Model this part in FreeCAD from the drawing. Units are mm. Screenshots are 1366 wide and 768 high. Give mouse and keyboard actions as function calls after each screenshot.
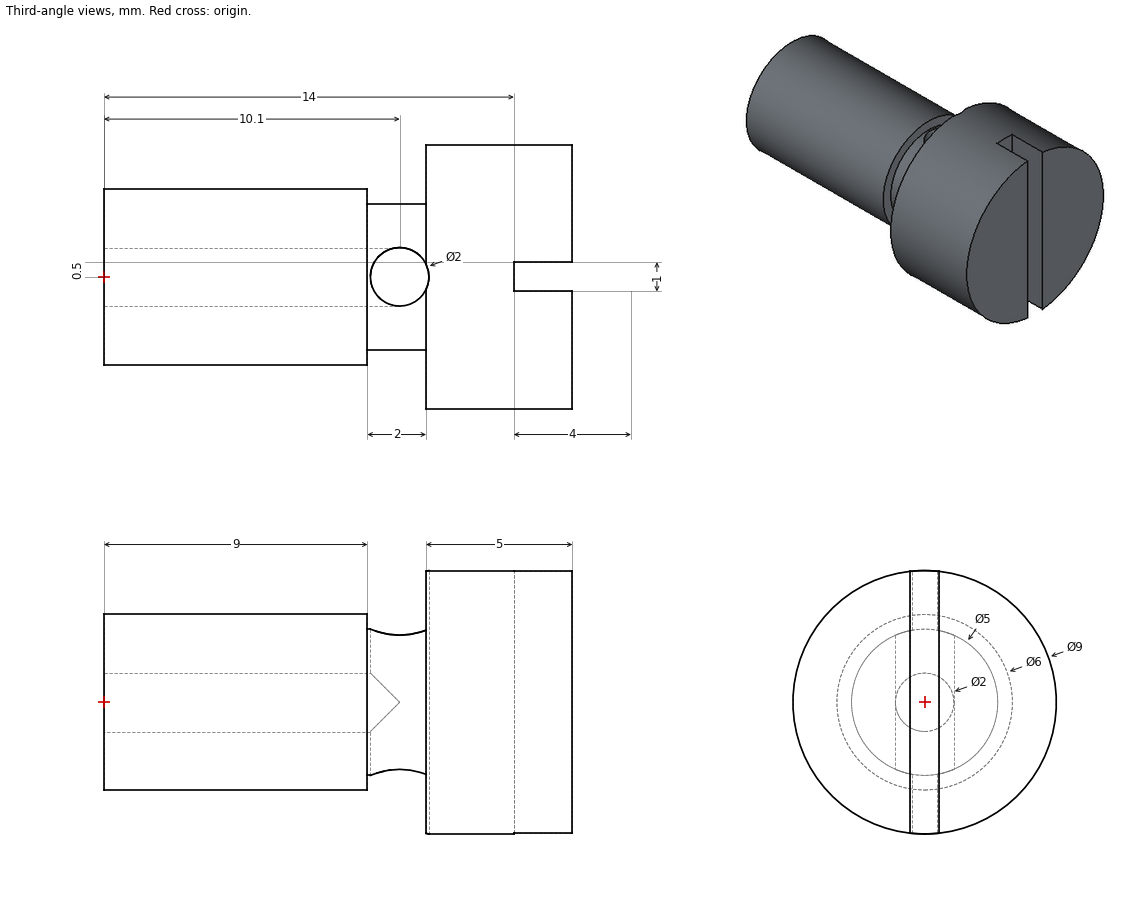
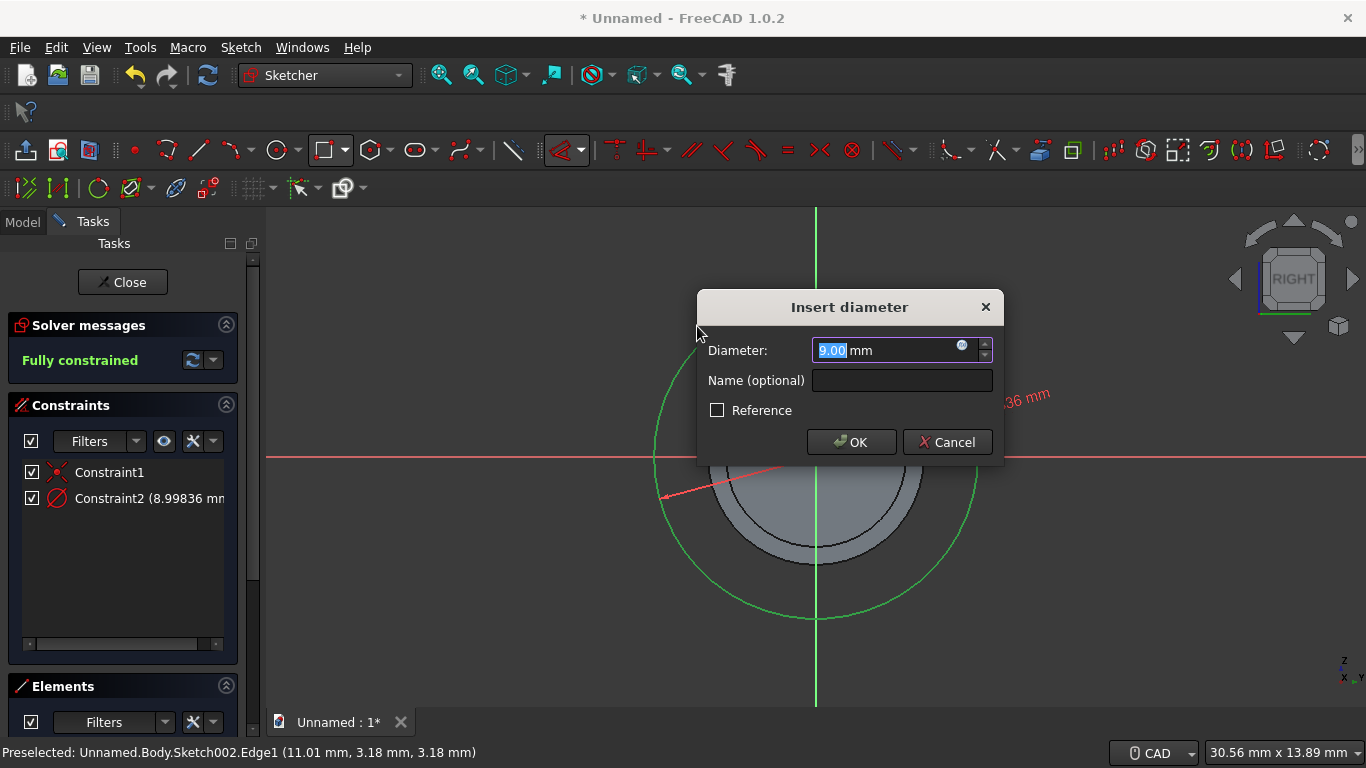
text(9)
key(Return)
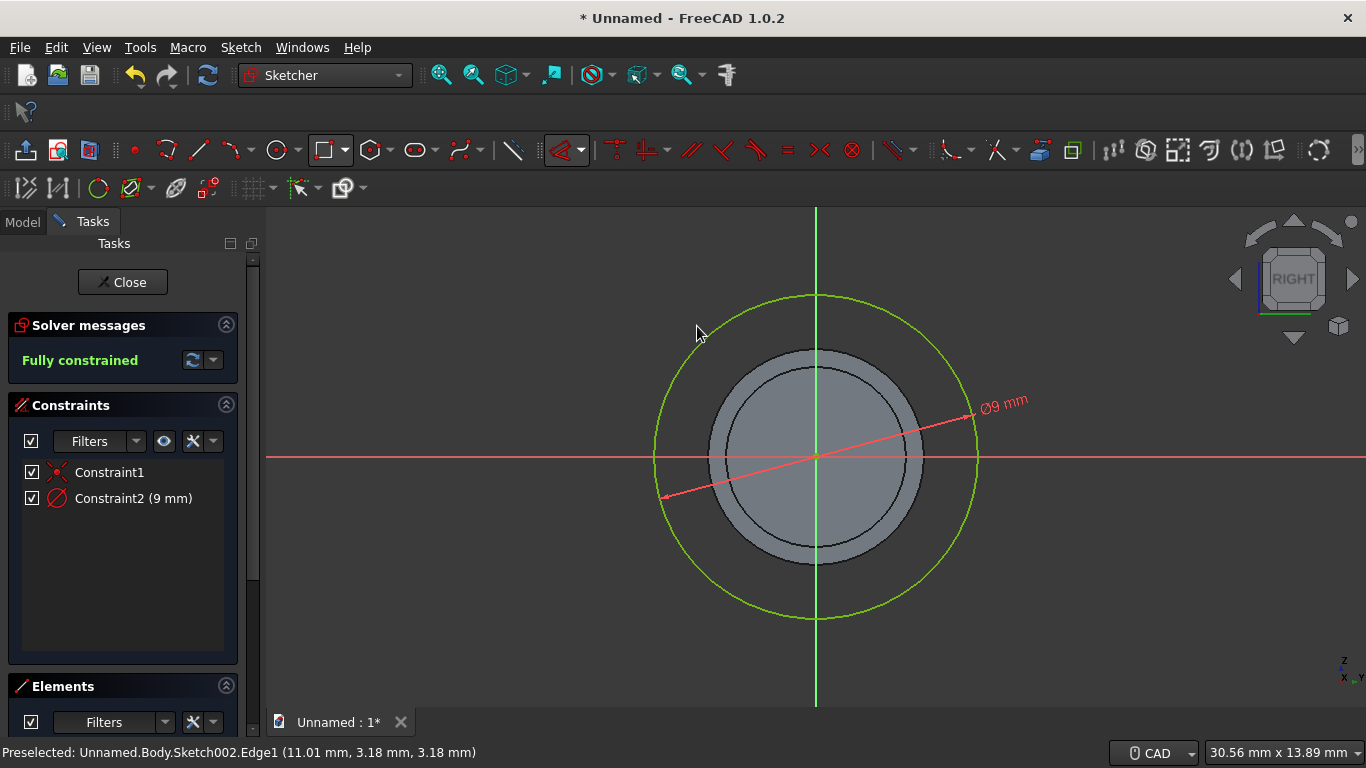
click(123, 282)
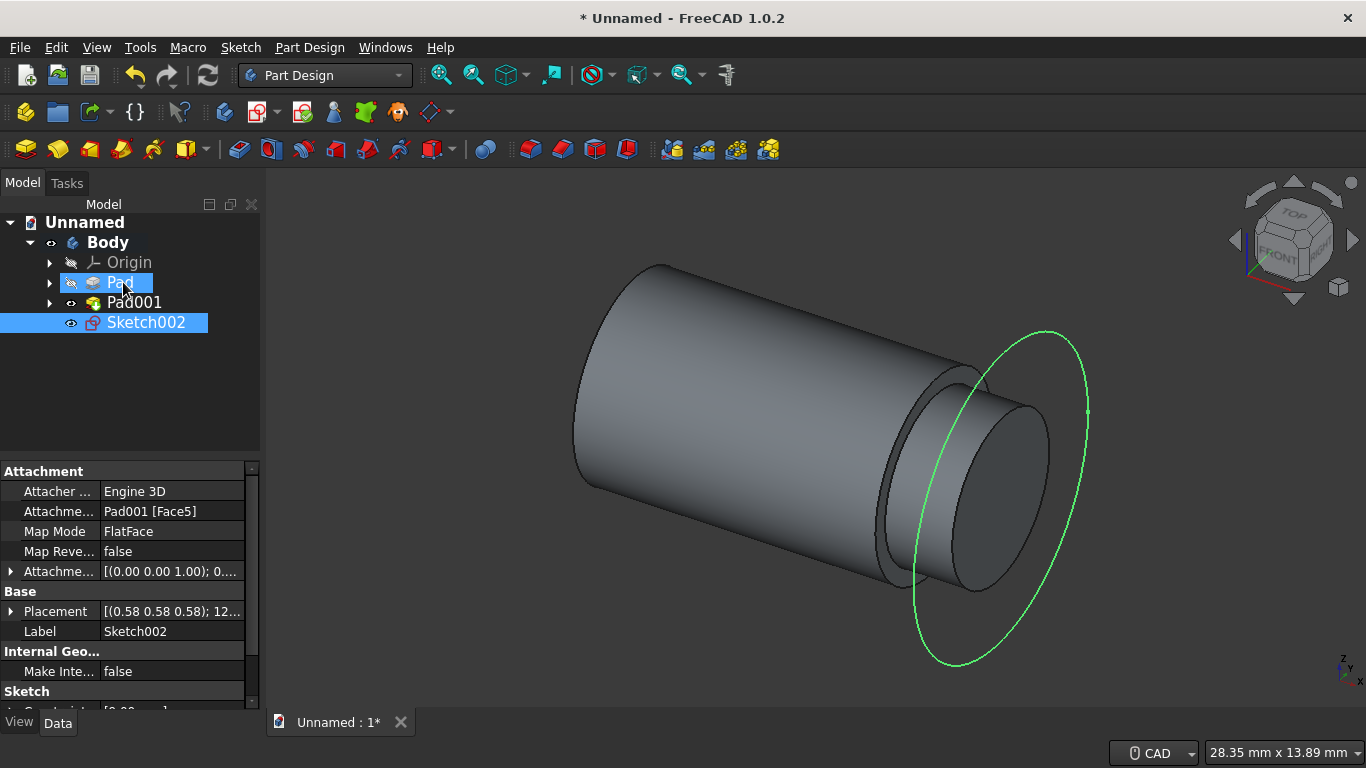
click(26, 150)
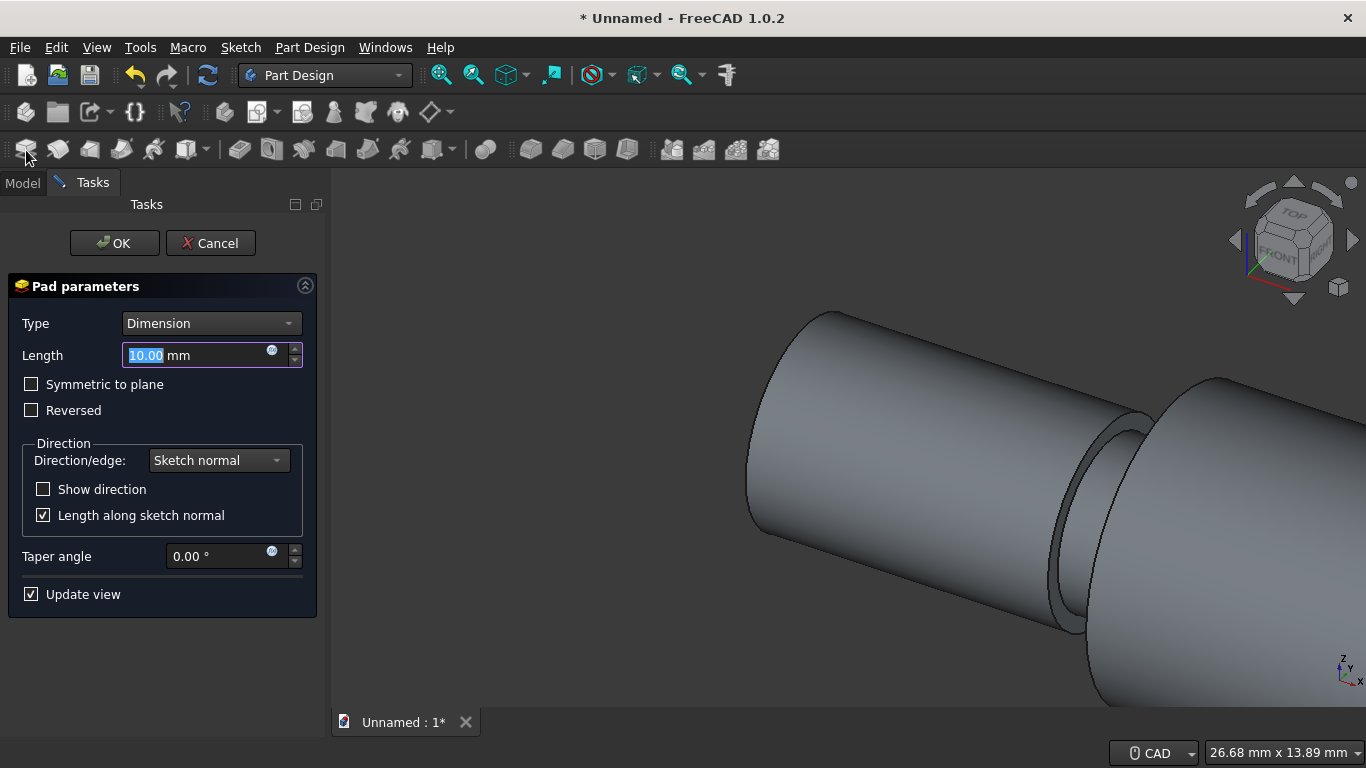
text(5)
key(Tab)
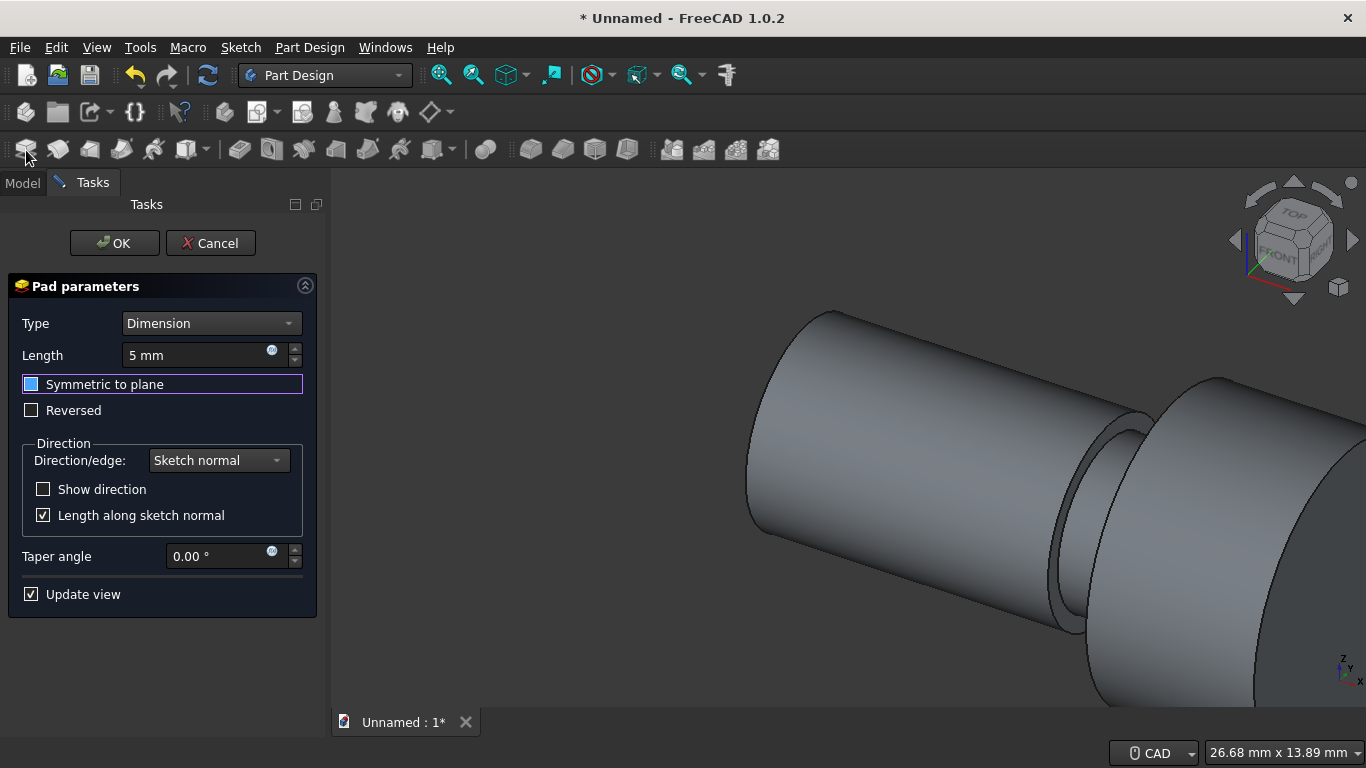
click(115, 243)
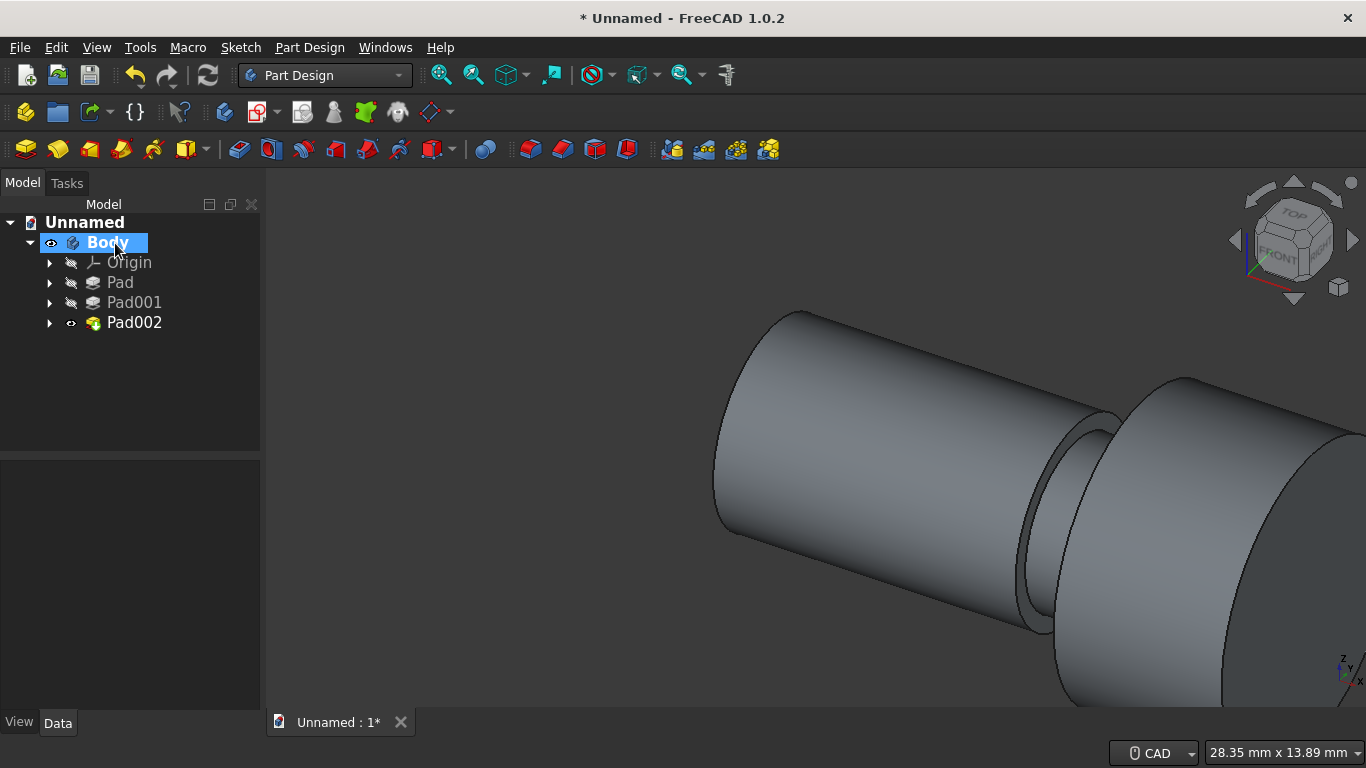
key(v)
key(f)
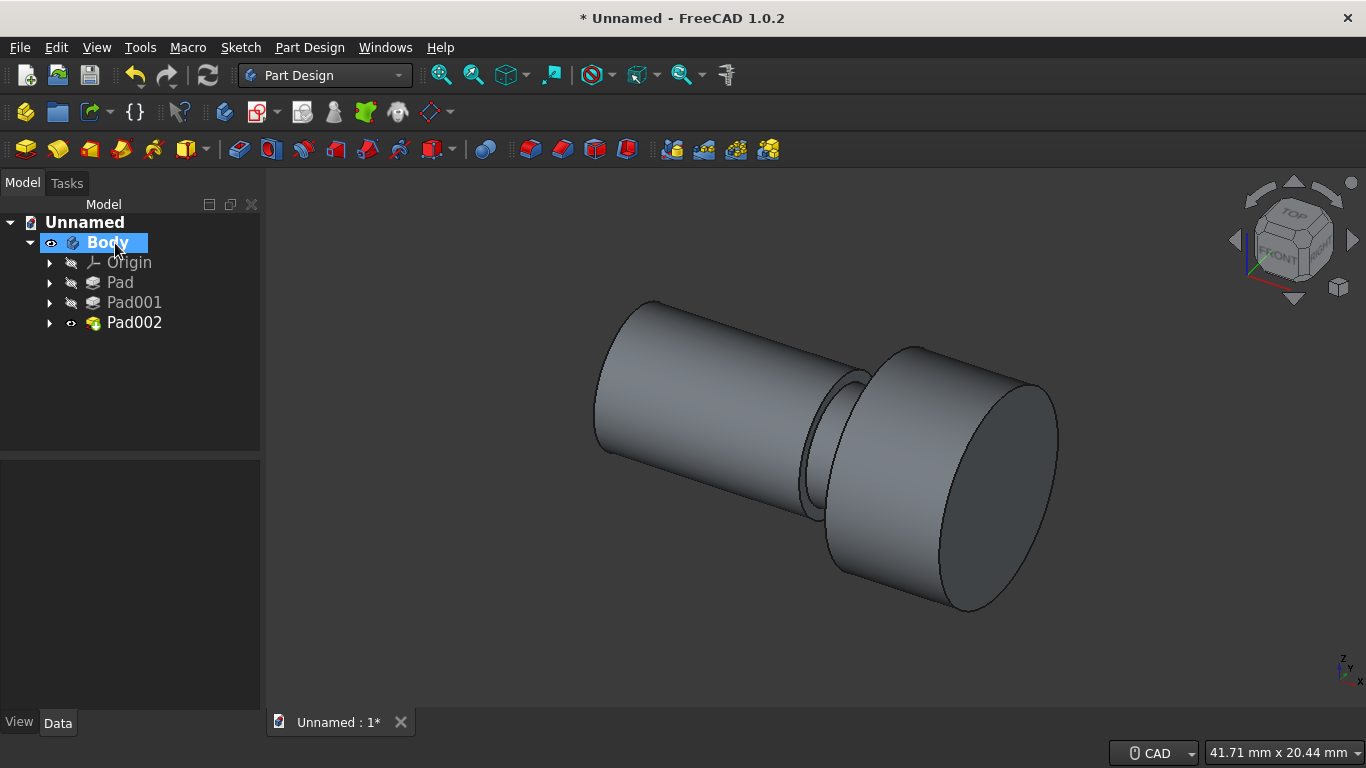
key(6)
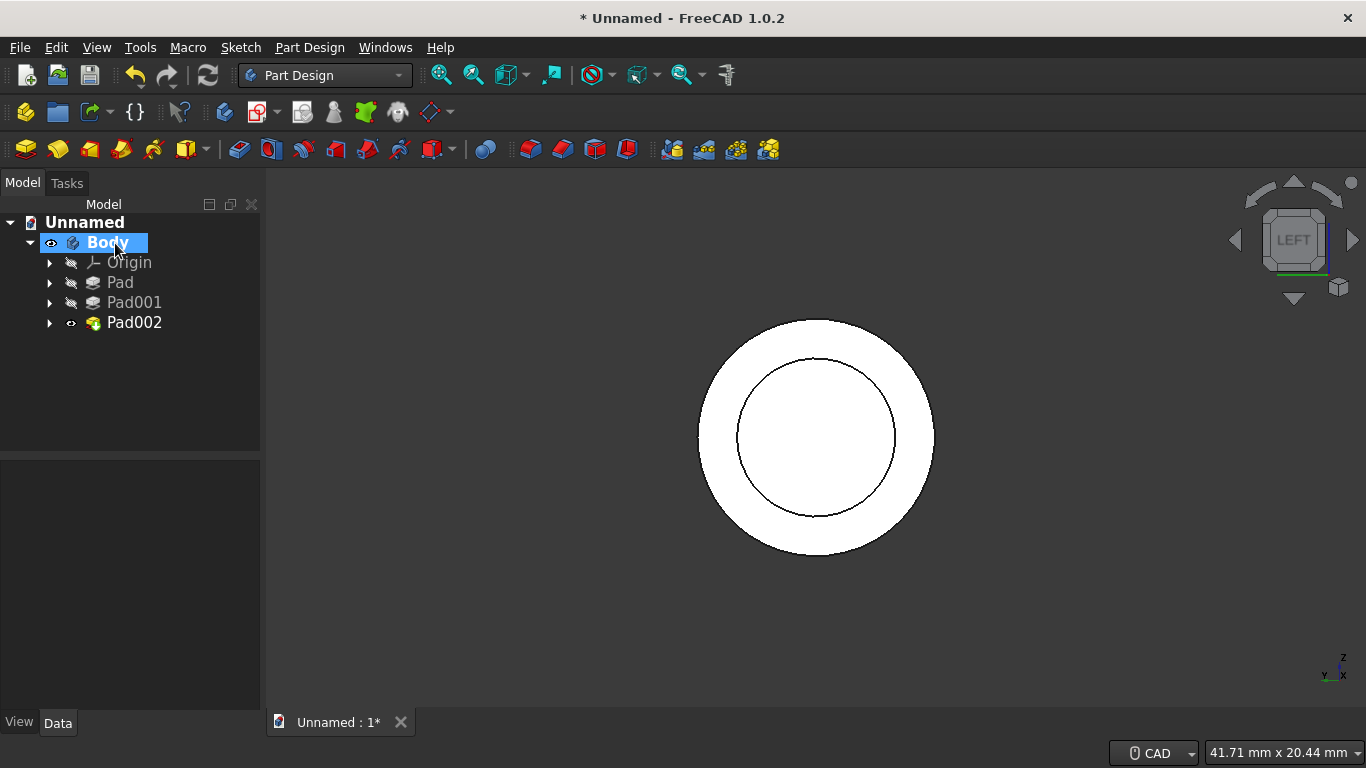
click(442, 76)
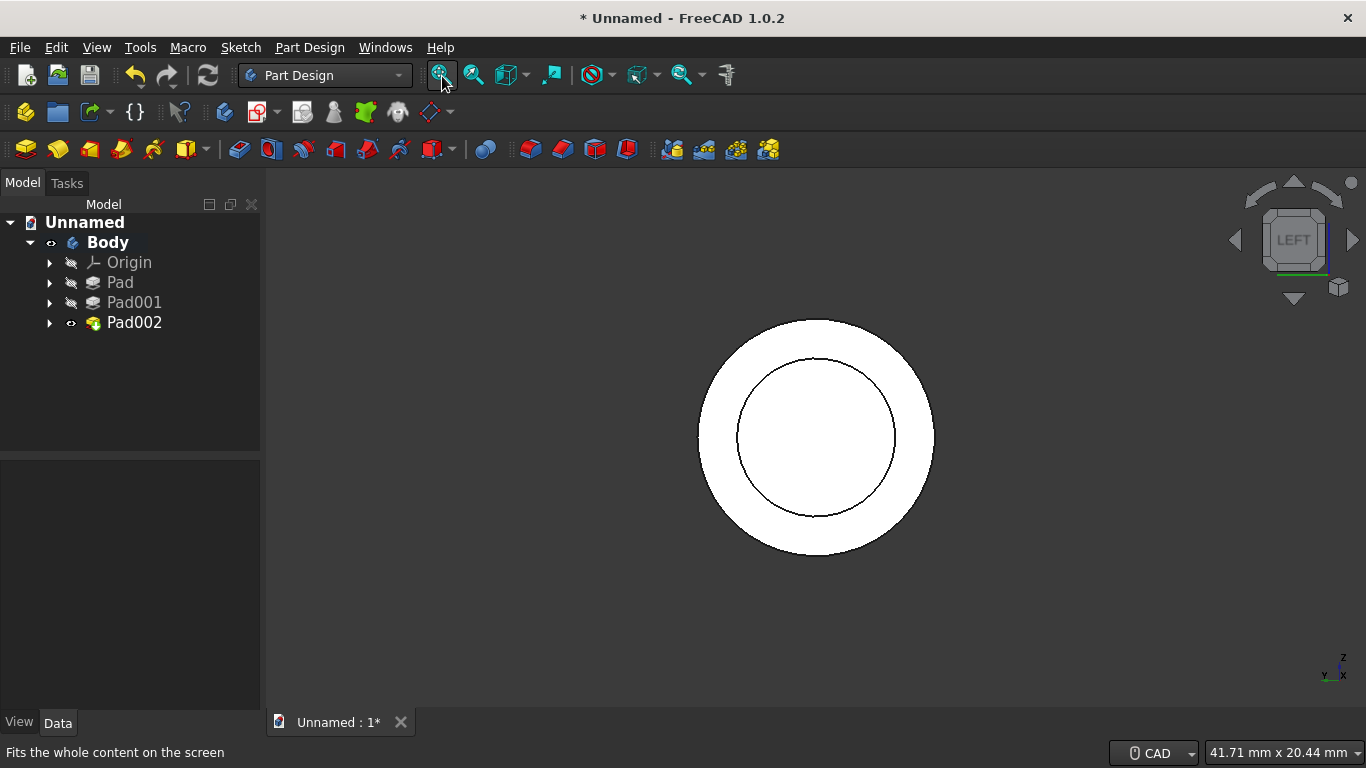
click(816, 436)